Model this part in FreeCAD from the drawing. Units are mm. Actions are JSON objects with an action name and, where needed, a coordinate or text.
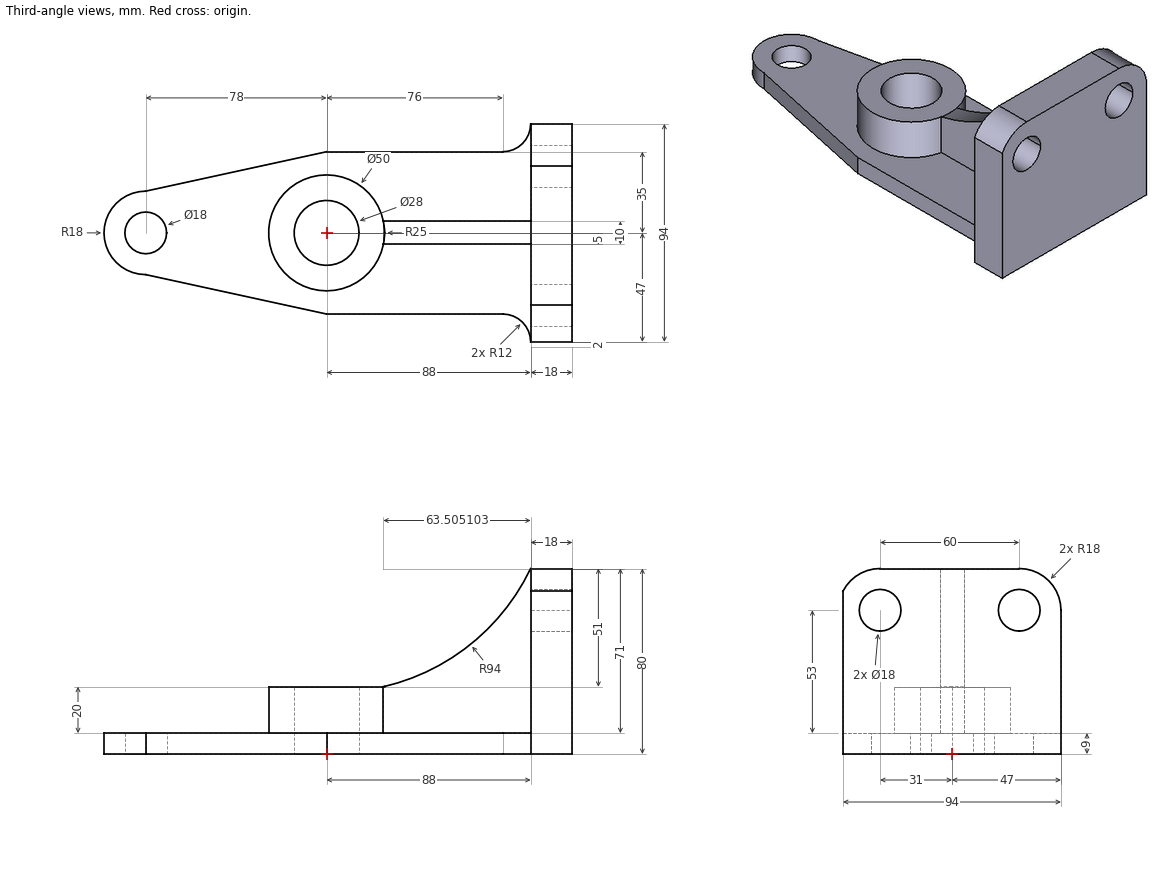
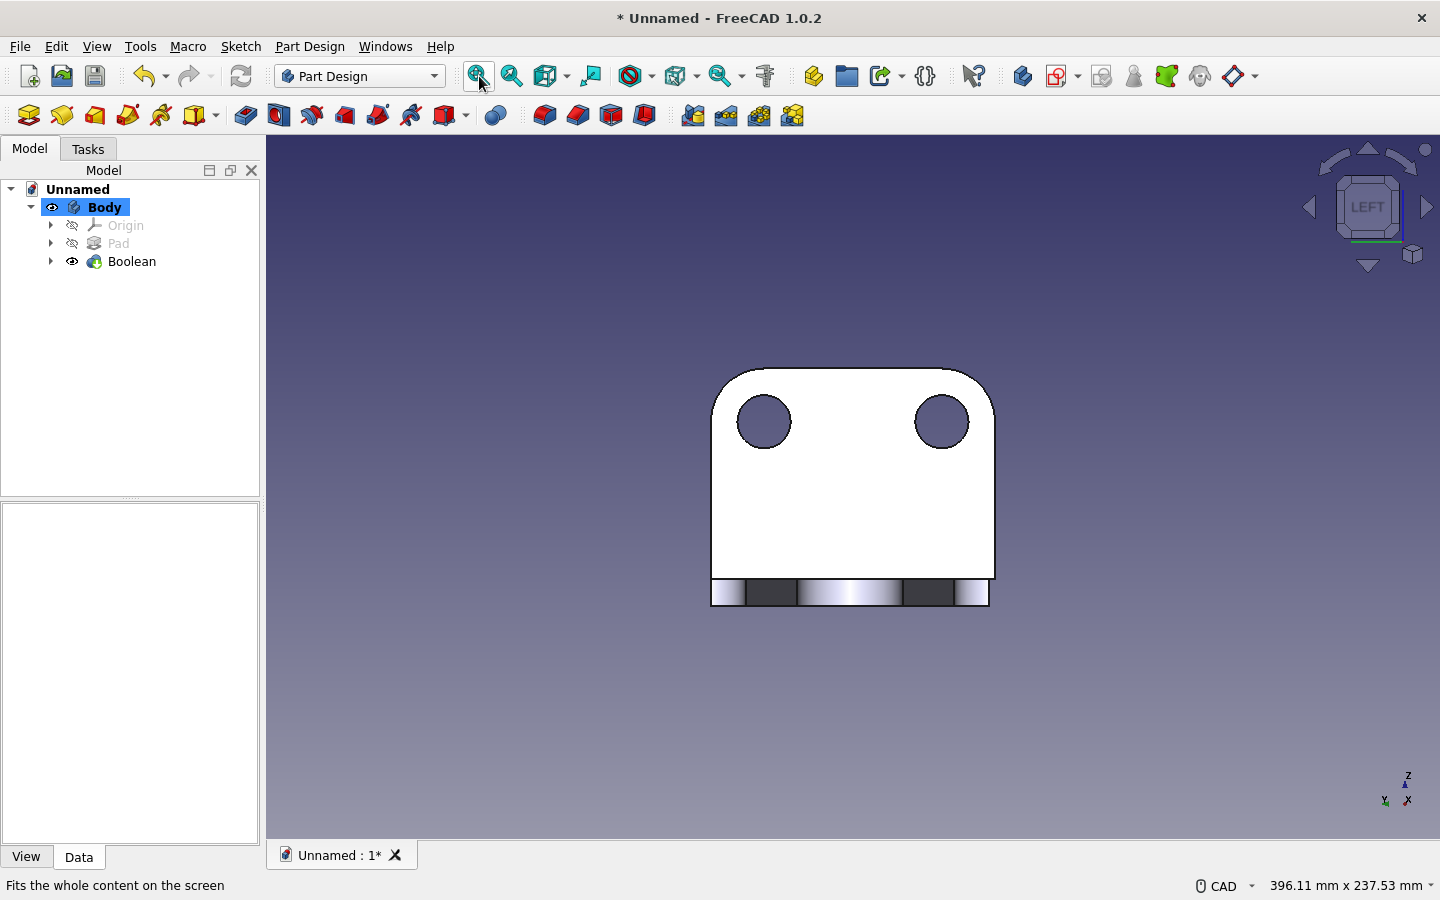
{"action": "left_click", "coordinate": [479, 76]}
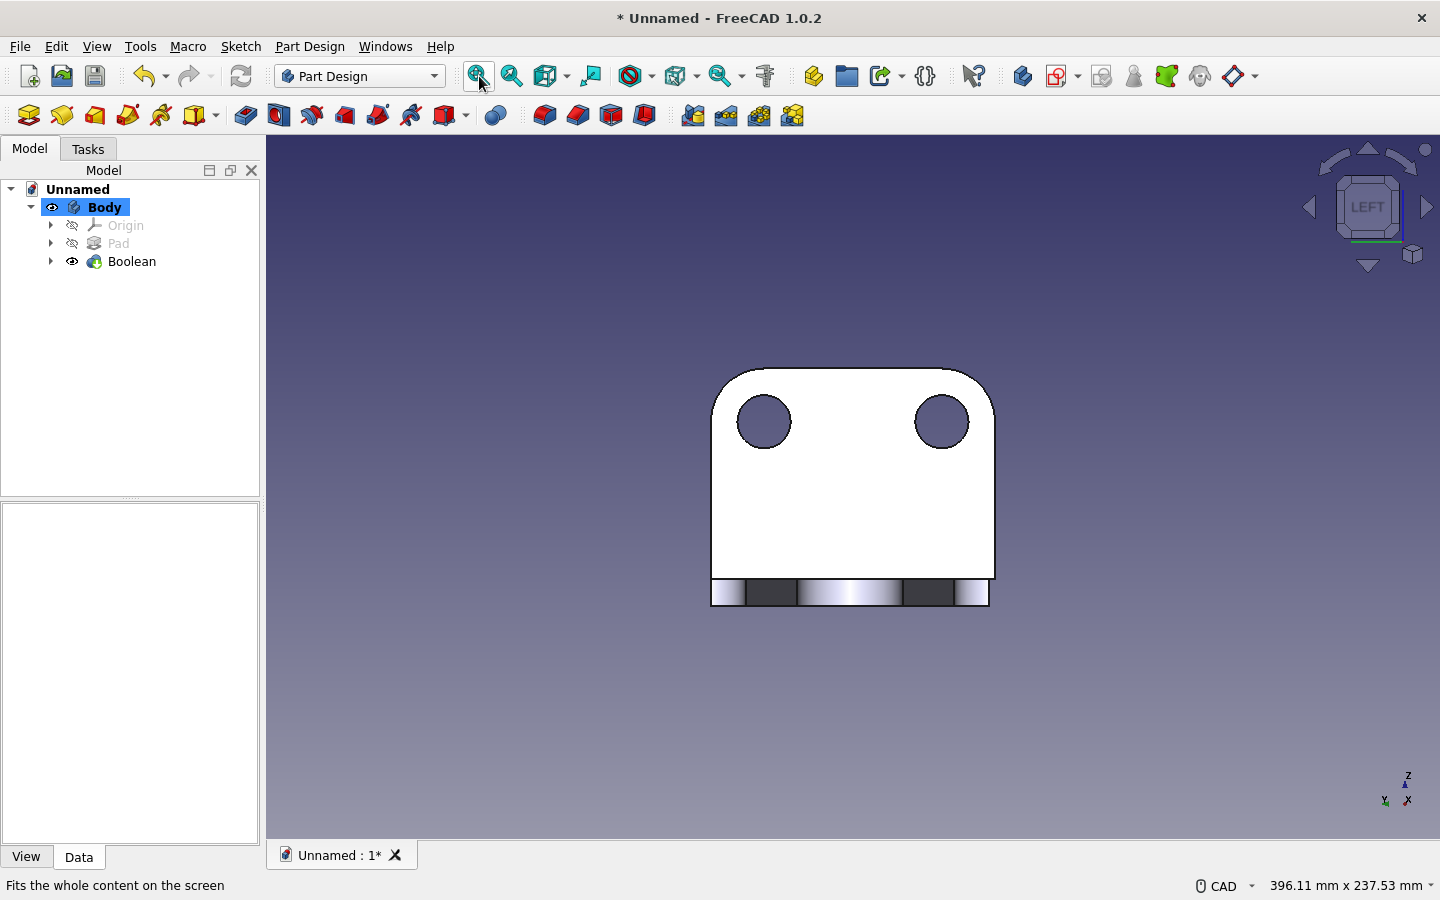
{"action": "left_click", "coordinate": [853, 473]}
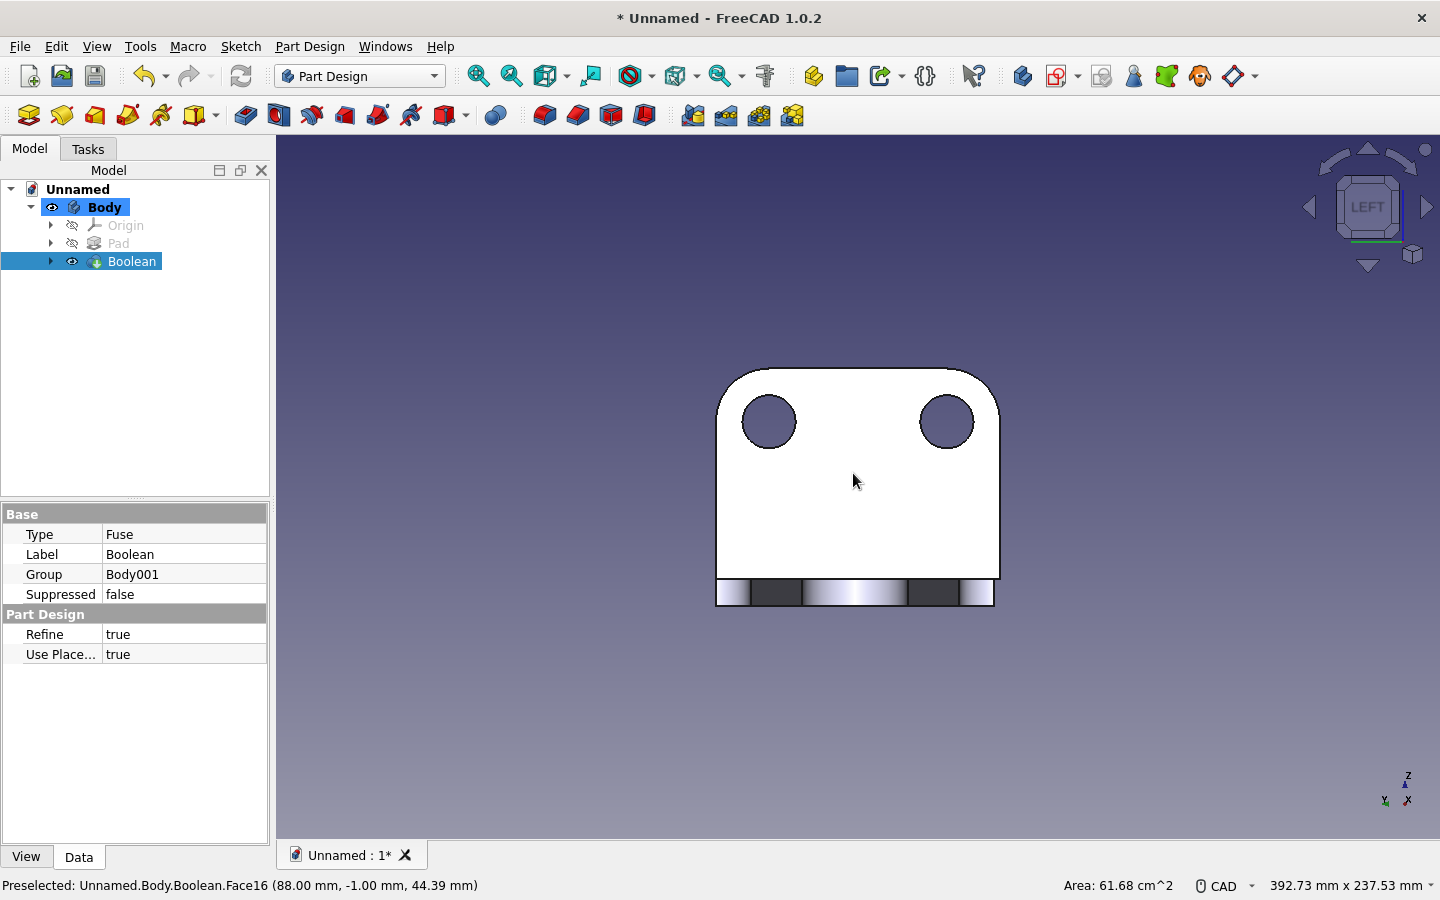
{"action": "left_click", "coordinate": [1056, 76]}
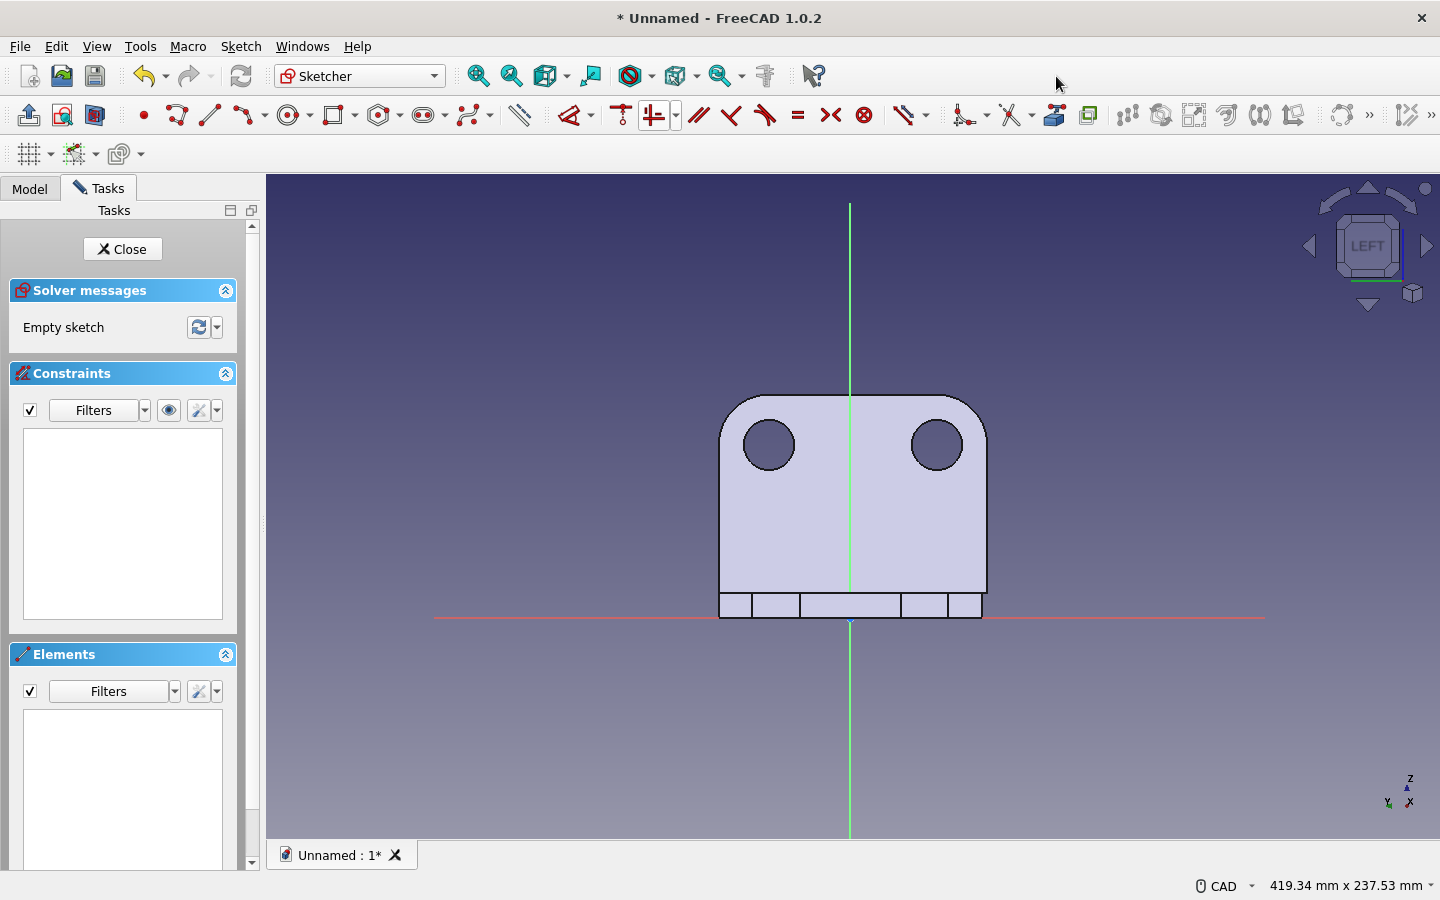
{"action": "key", "text": "q s"}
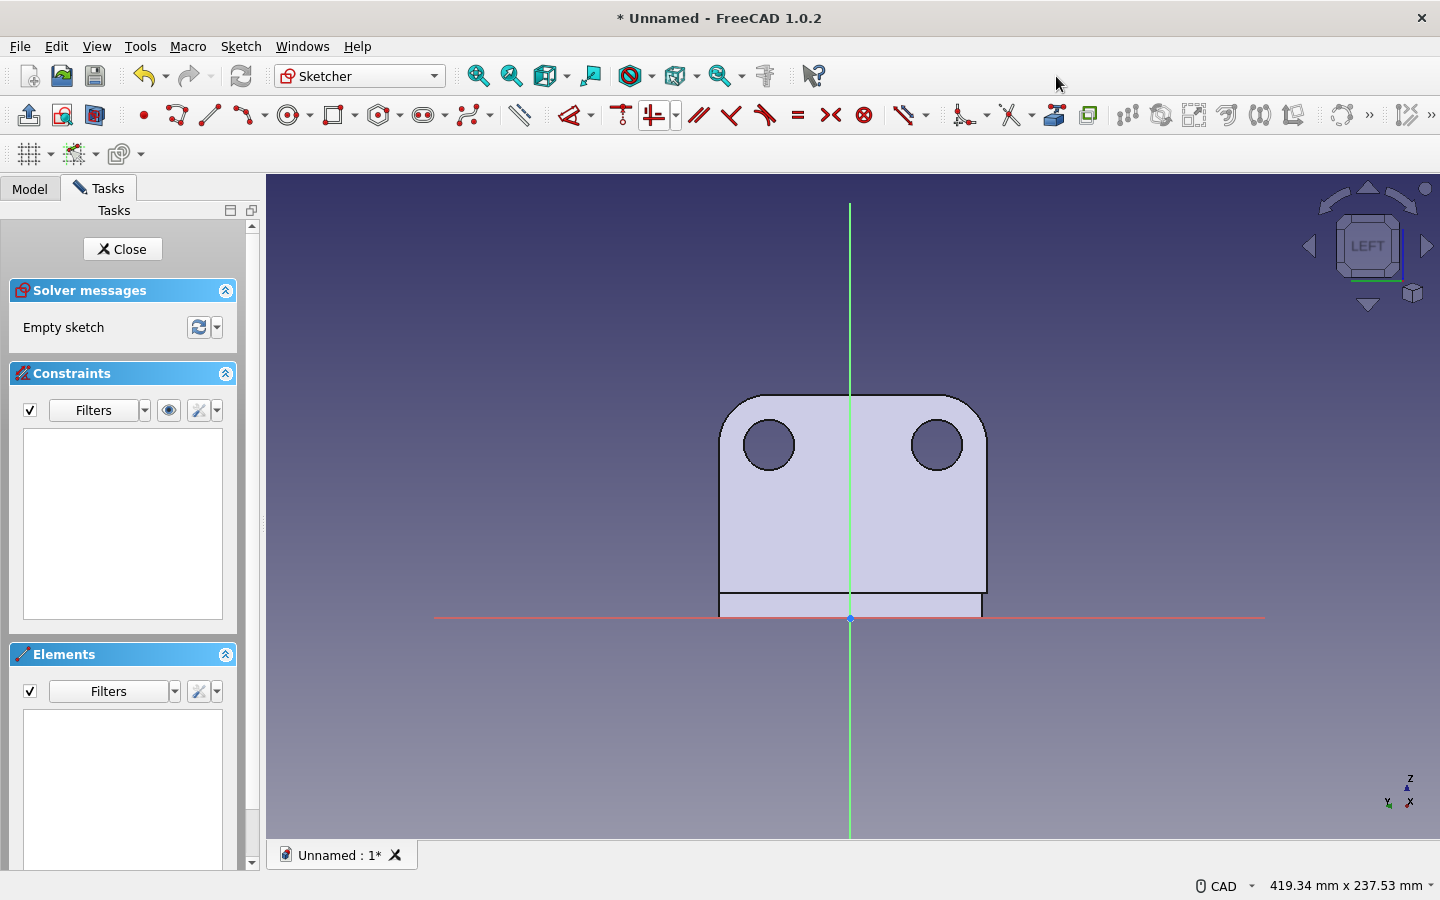
{"action": "scroll", "coordinate": [888, 664], "scroll_direction": "up", "scroll_amount": 5}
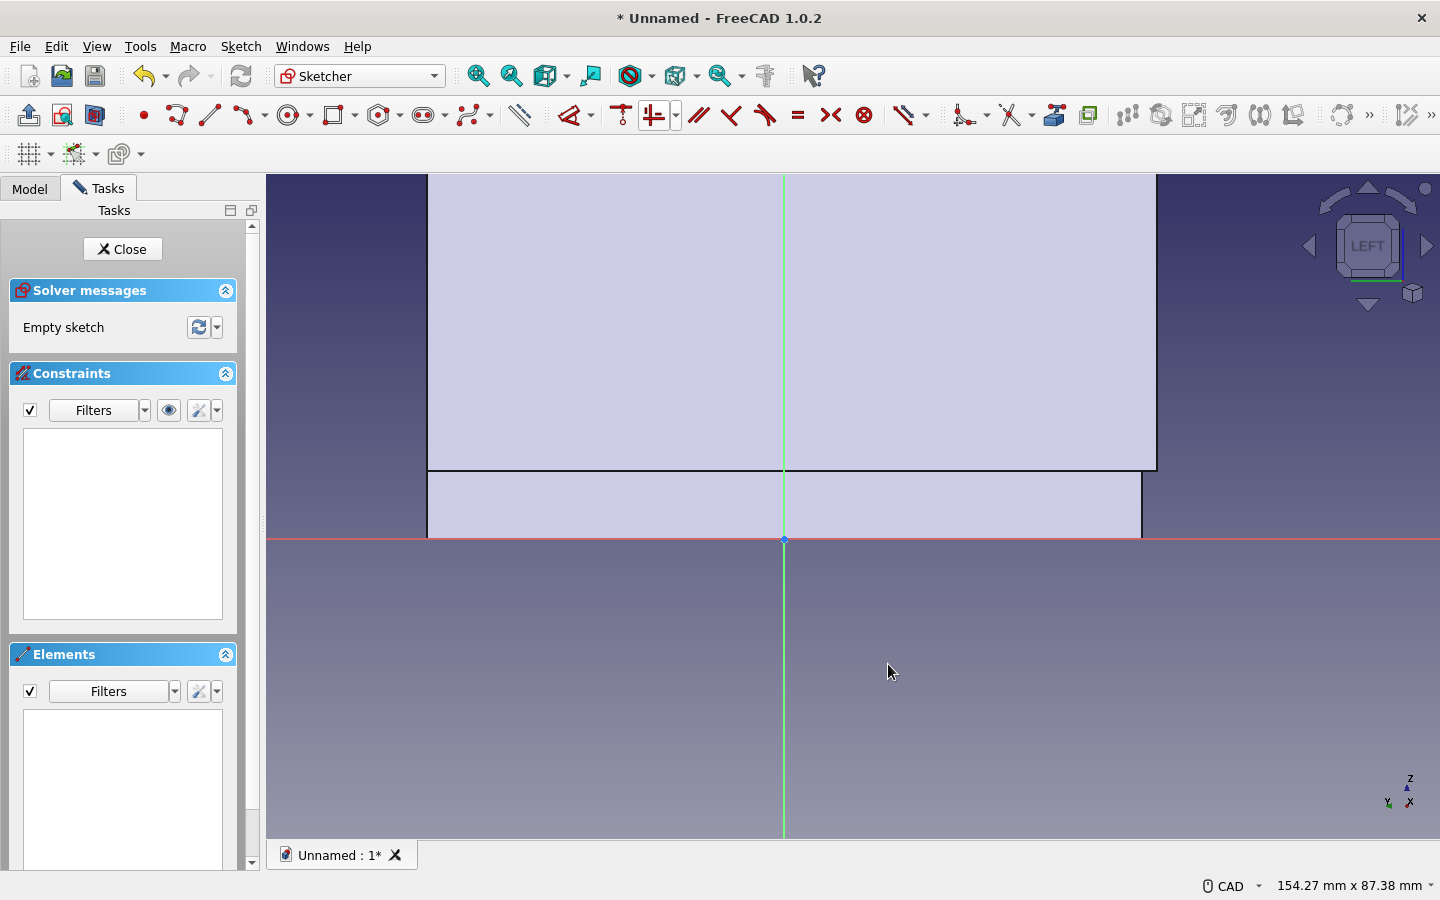
{"action": "left_click", "coordinate": [332, 116]}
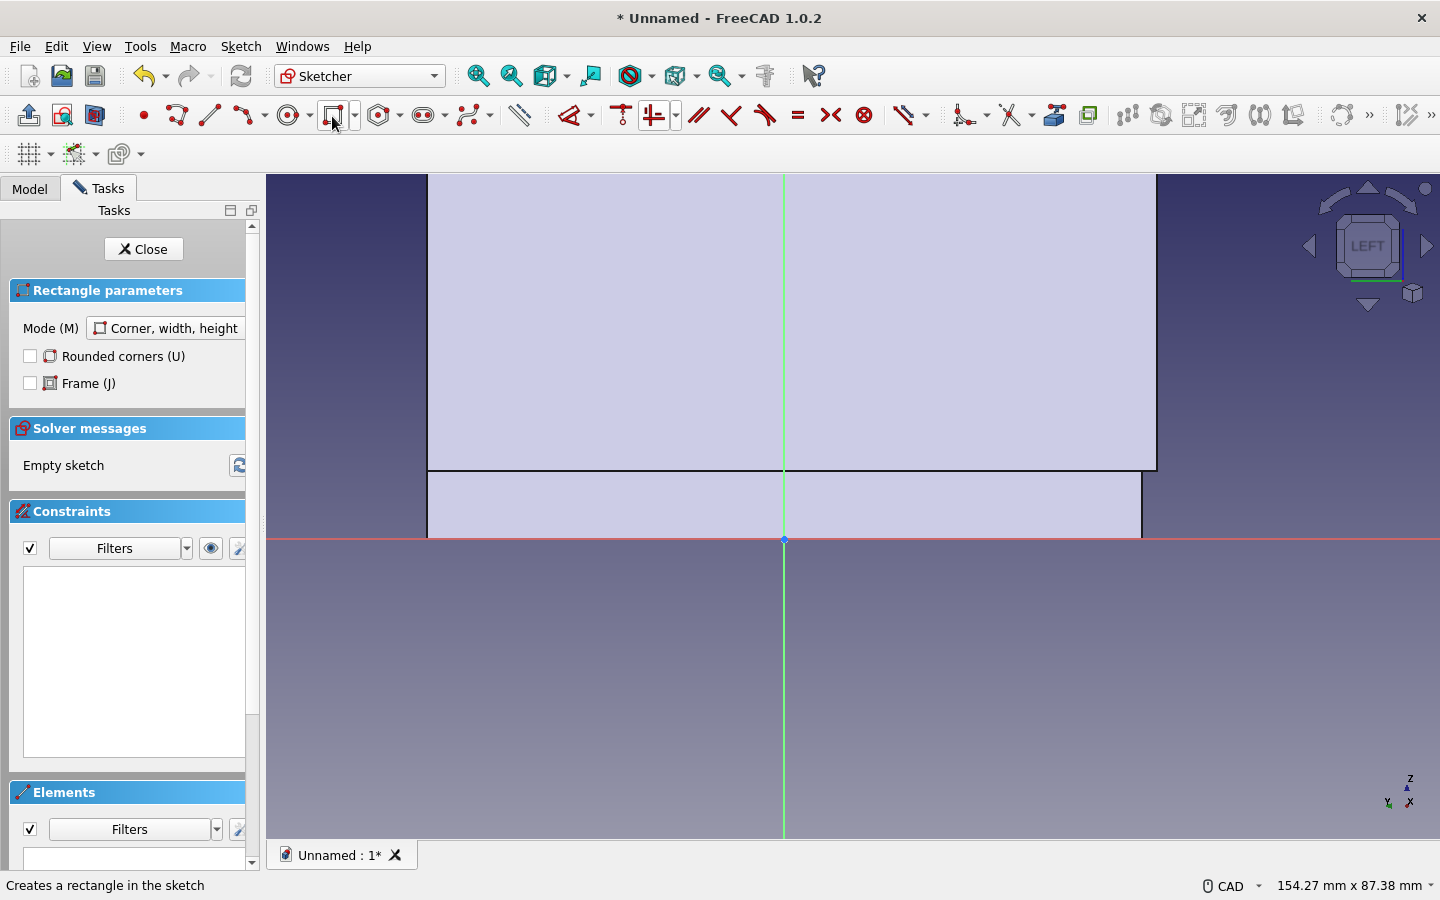
{"action": "left_click", "coordinate": [427, 471]}
{"action": "left_click", "coordinate": [1142, 539]}
{"action": "key", "text": "Escape"}